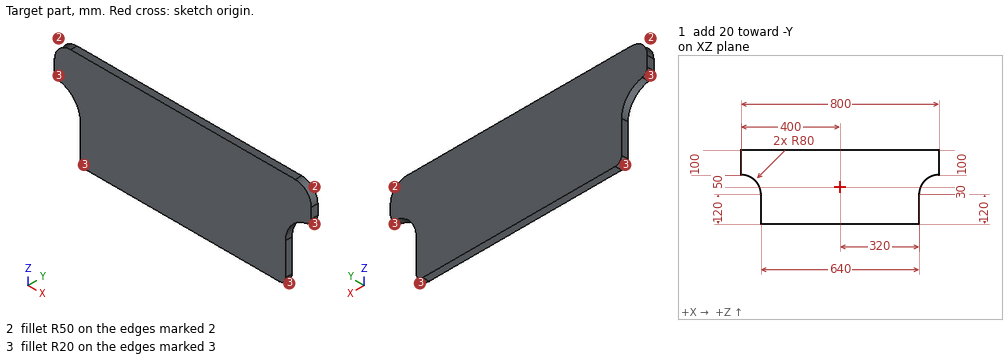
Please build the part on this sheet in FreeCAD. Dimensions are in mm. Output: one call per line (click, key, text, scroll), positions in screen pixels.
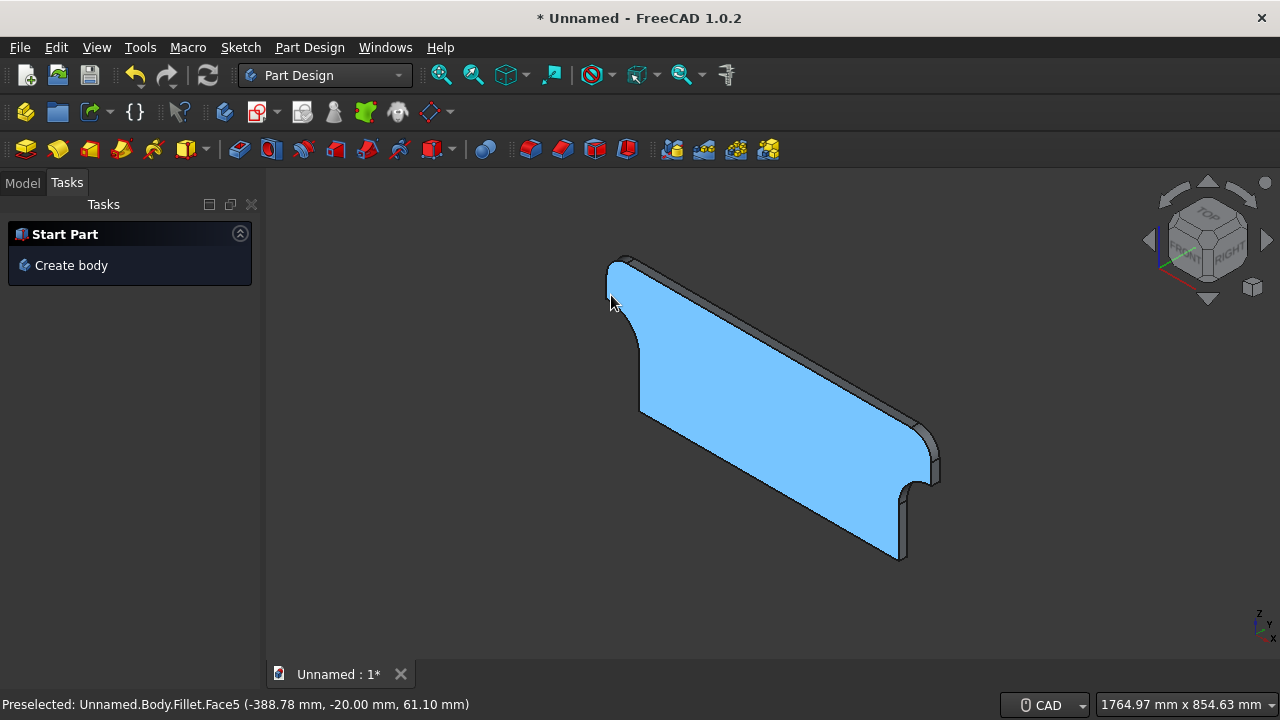
key(2)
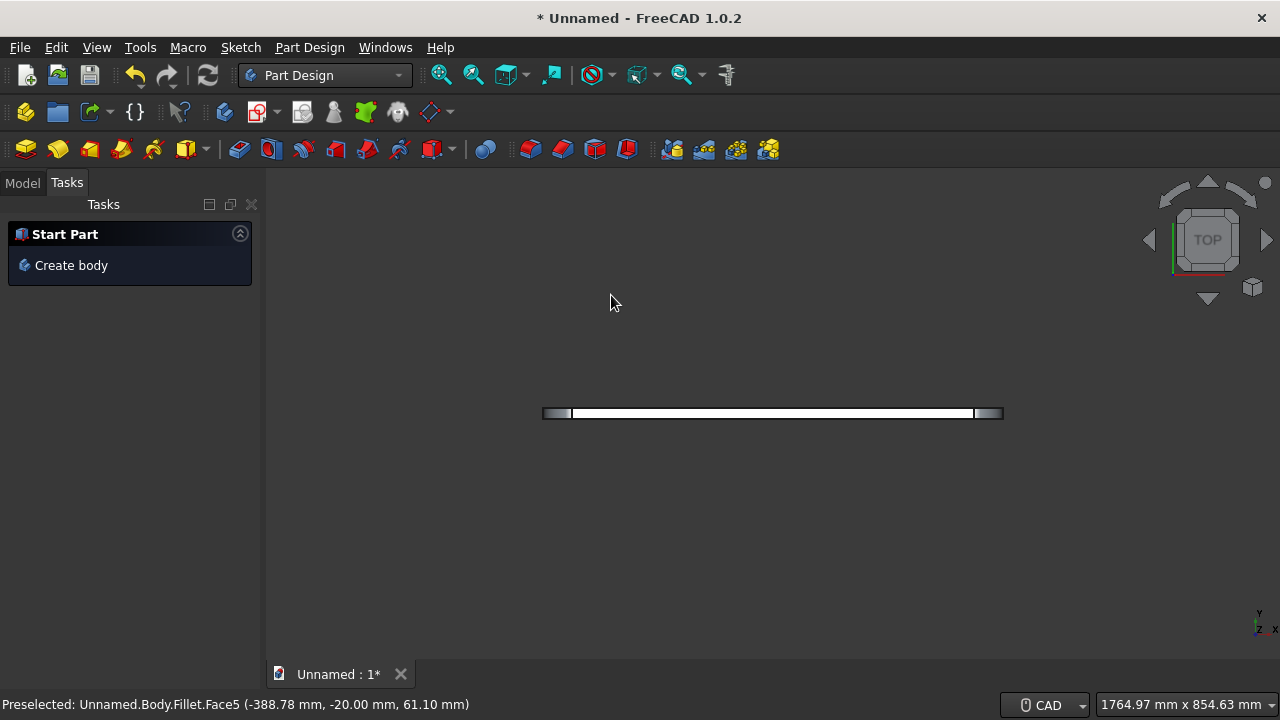
scroll(543, 412, up, 7)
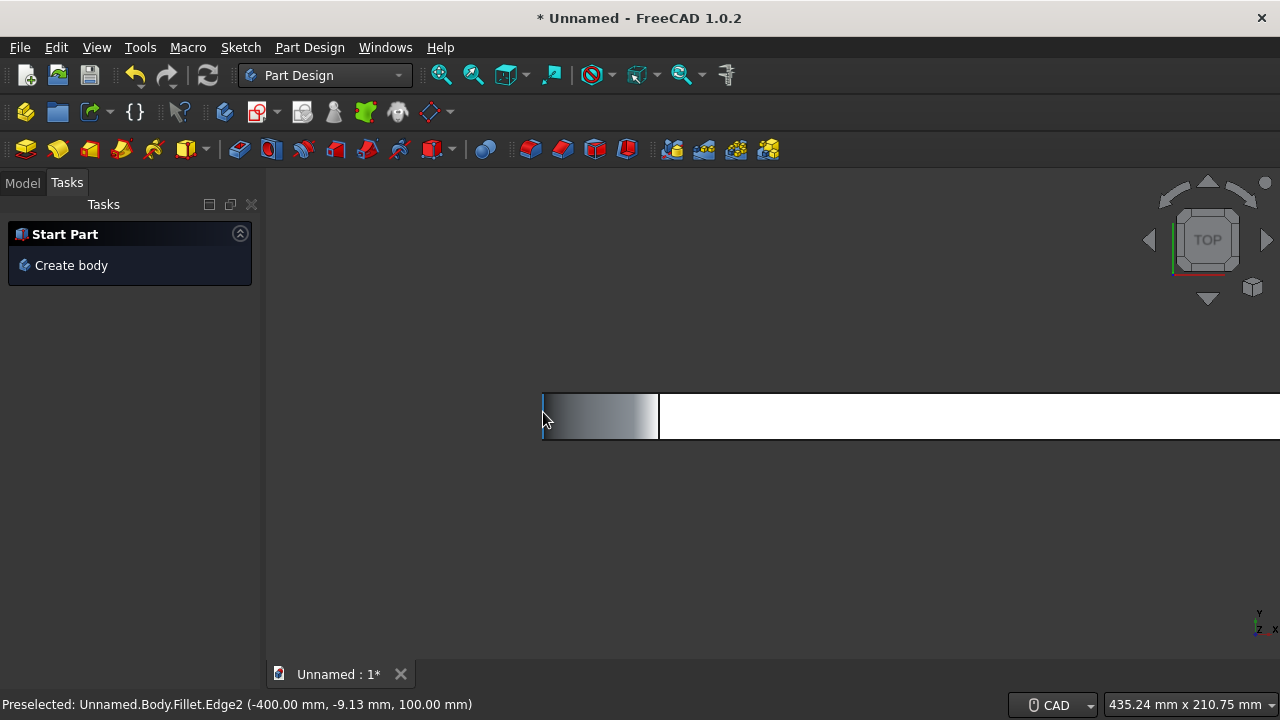
key(v)
key(f)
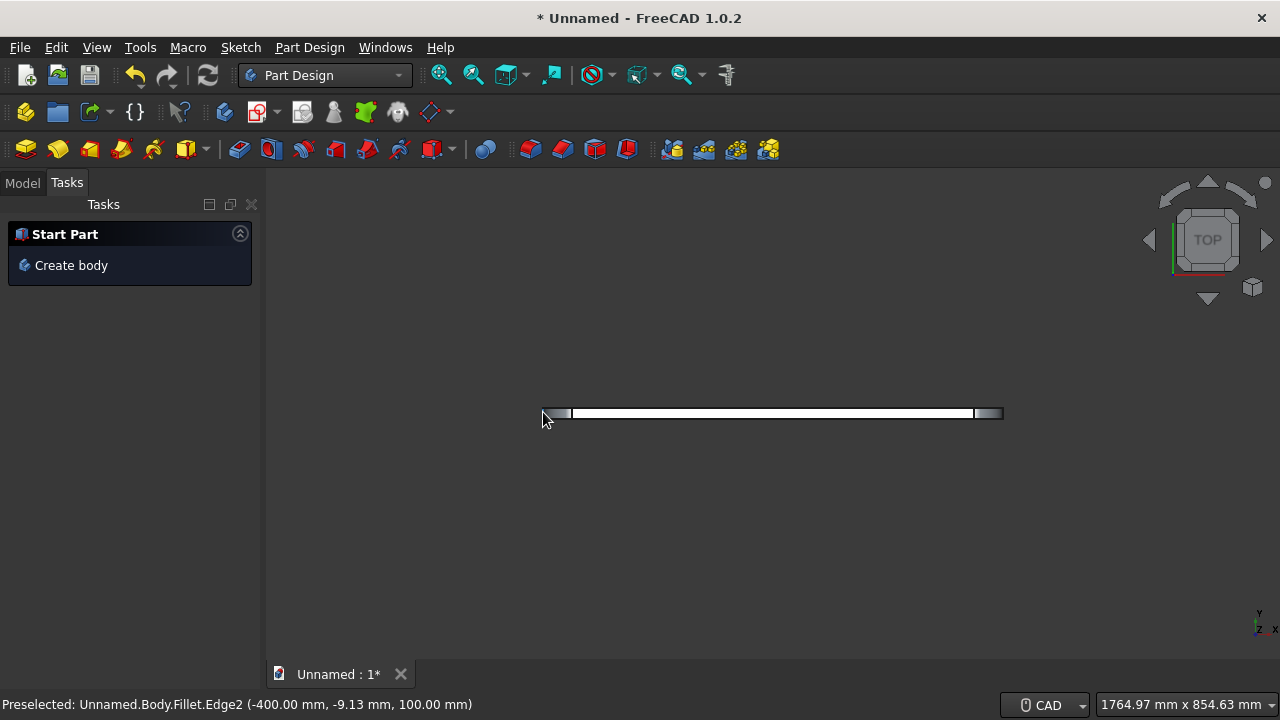
key(1)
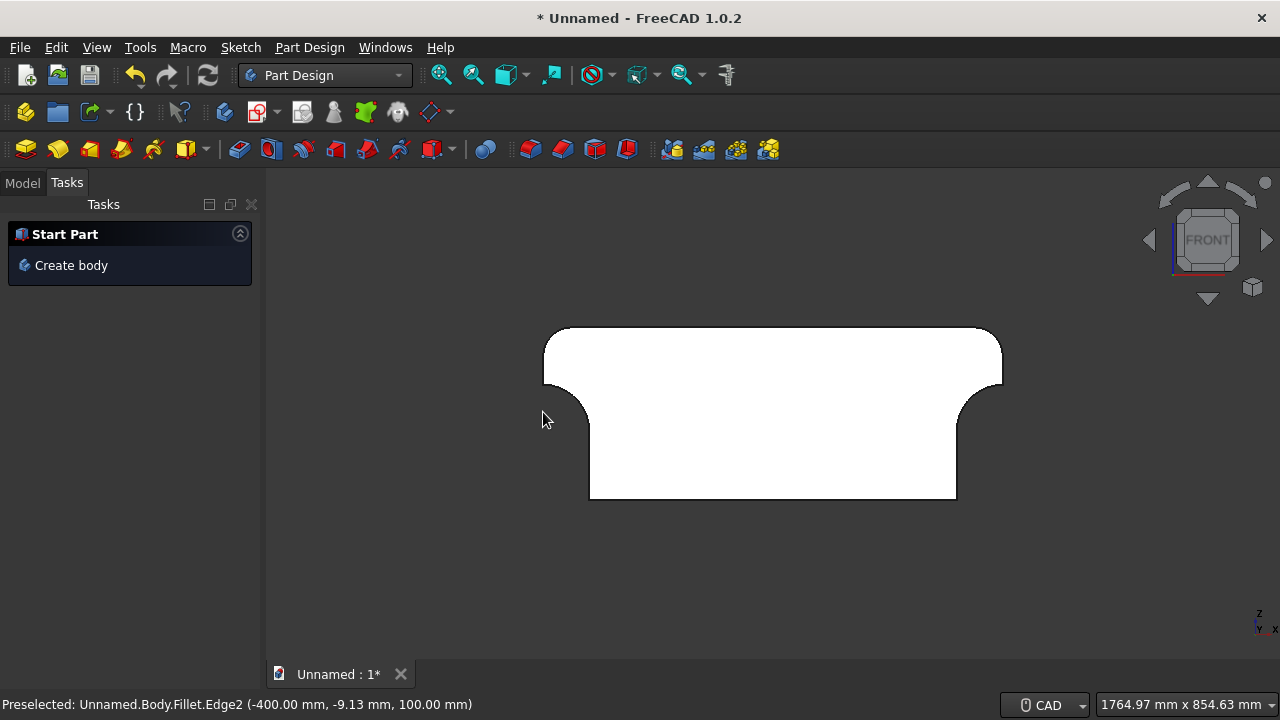
scroll(543, 384, up, 7)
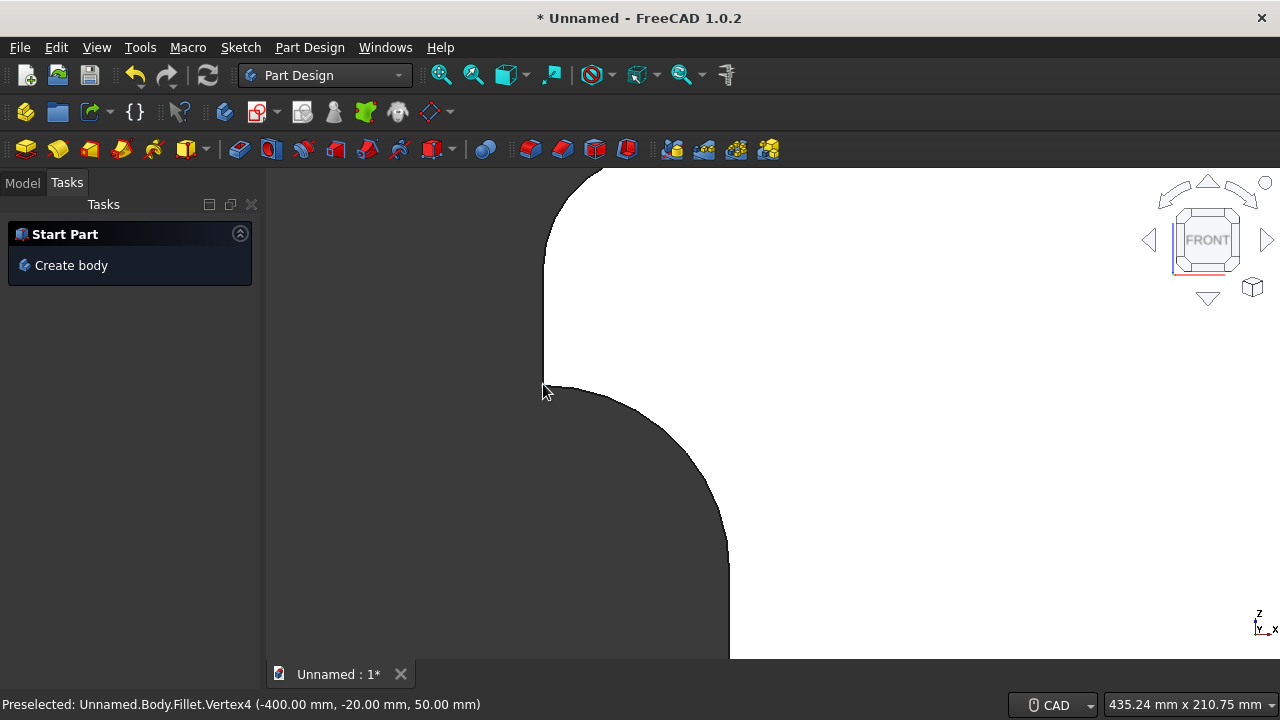
click(442, 76)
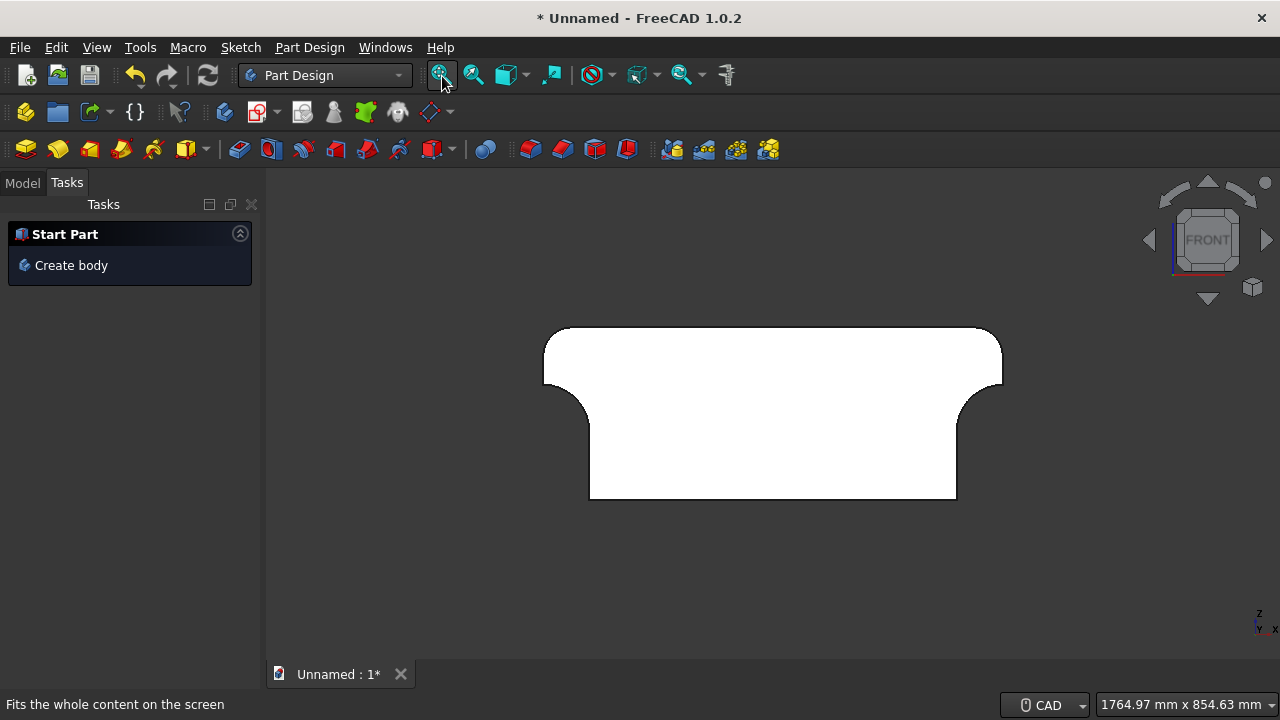
key(3)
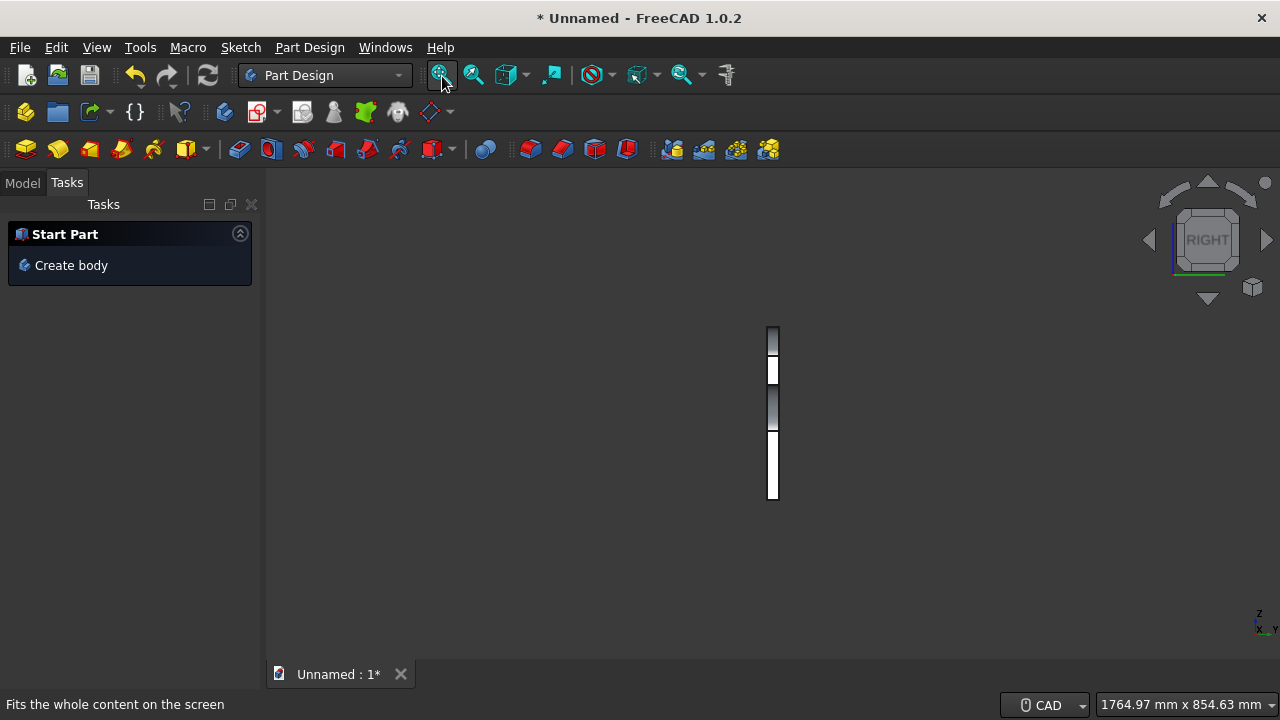
click(442, 76)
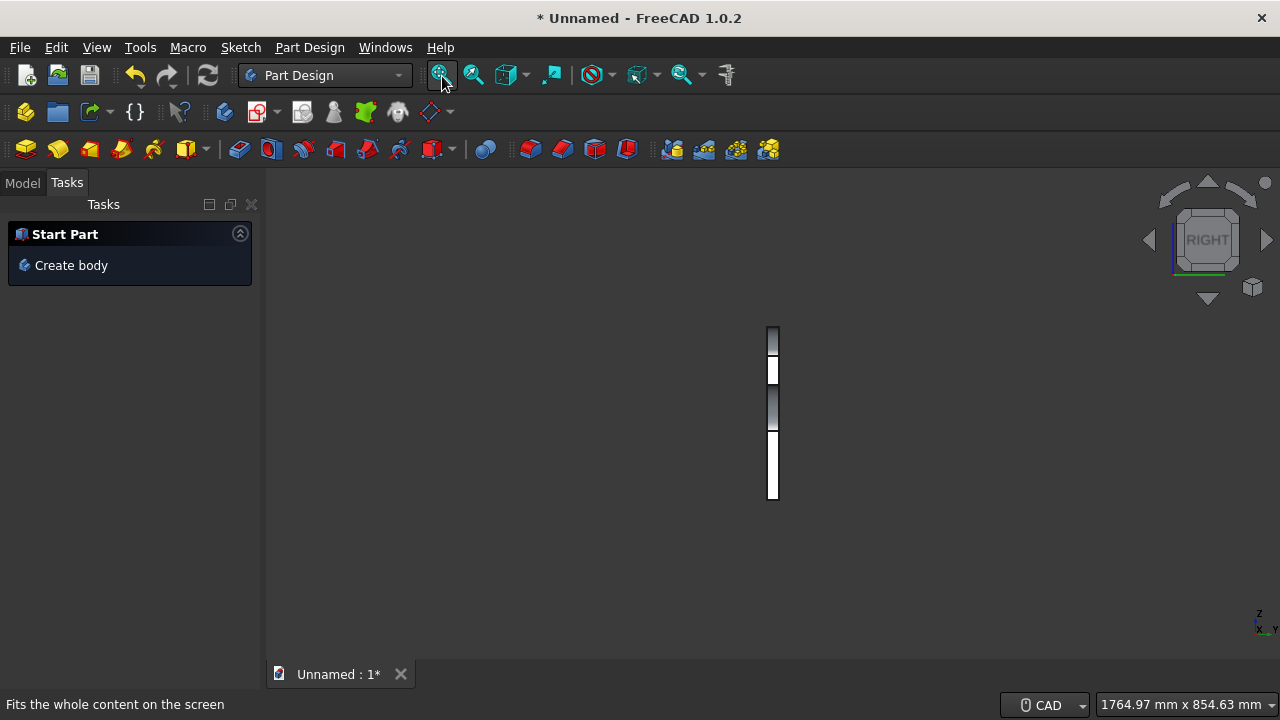
scroll(773, 384, up, 7)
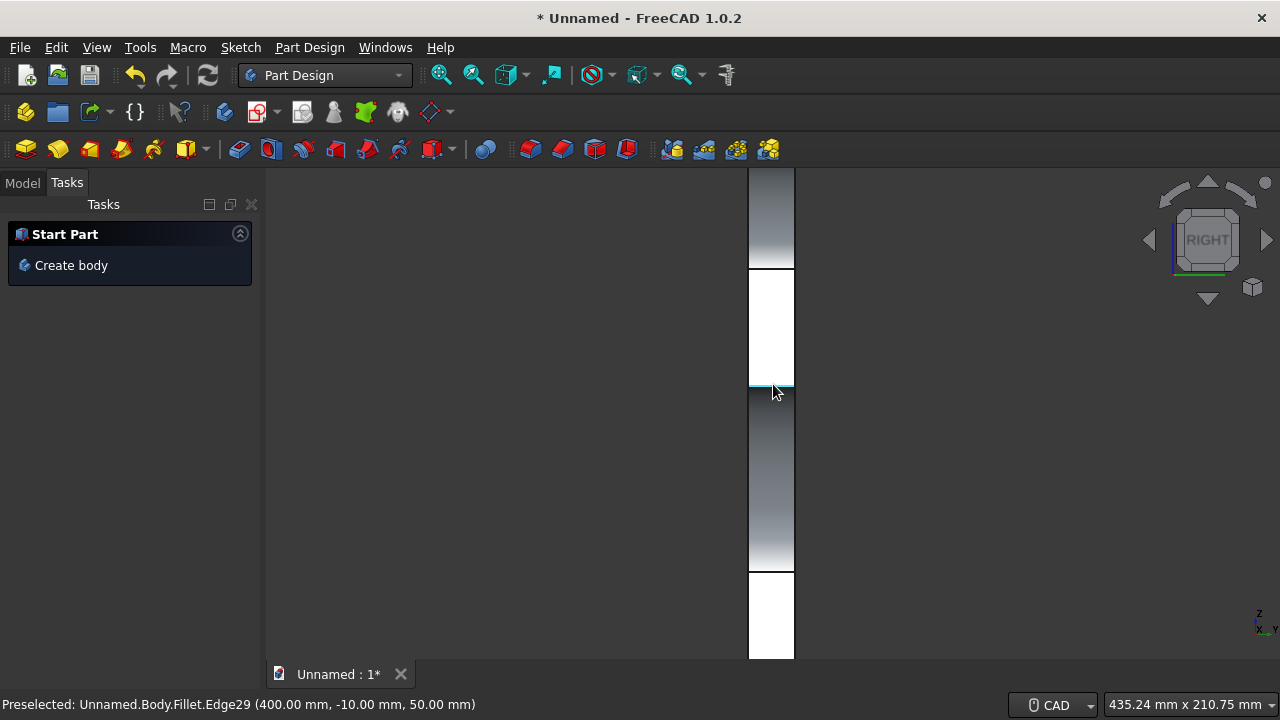
click(771, 385)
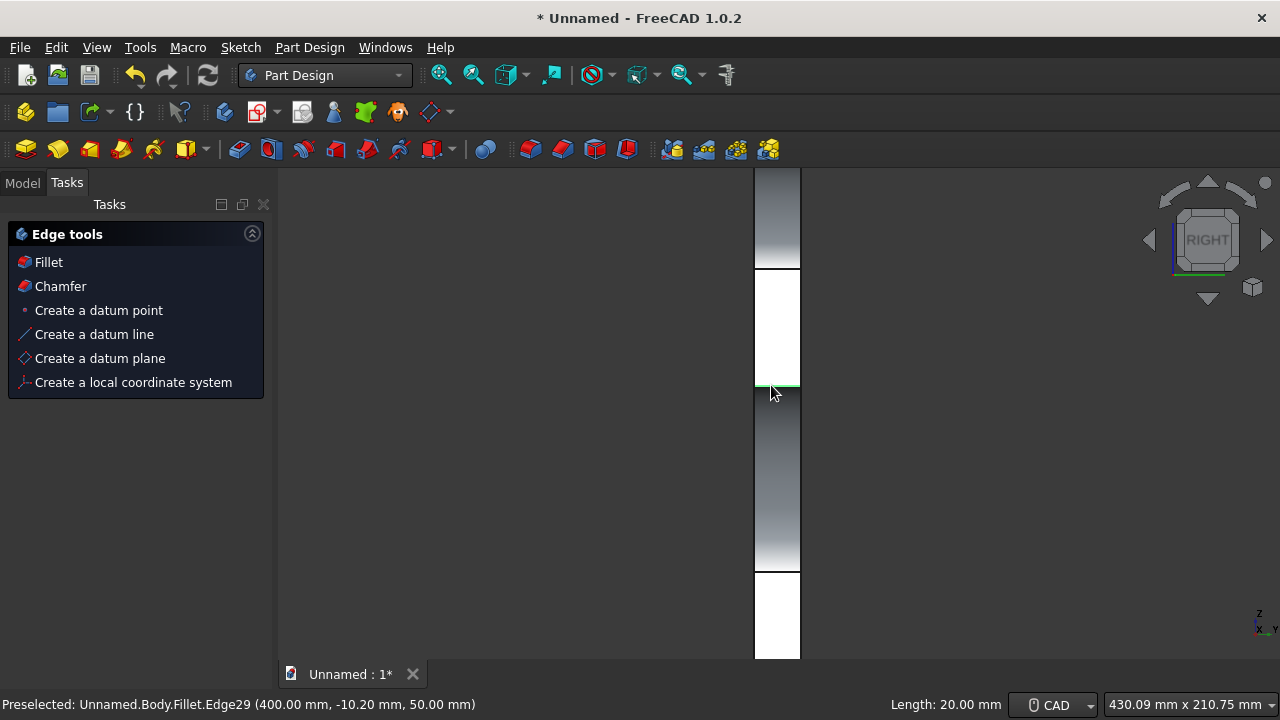
click(442, 76)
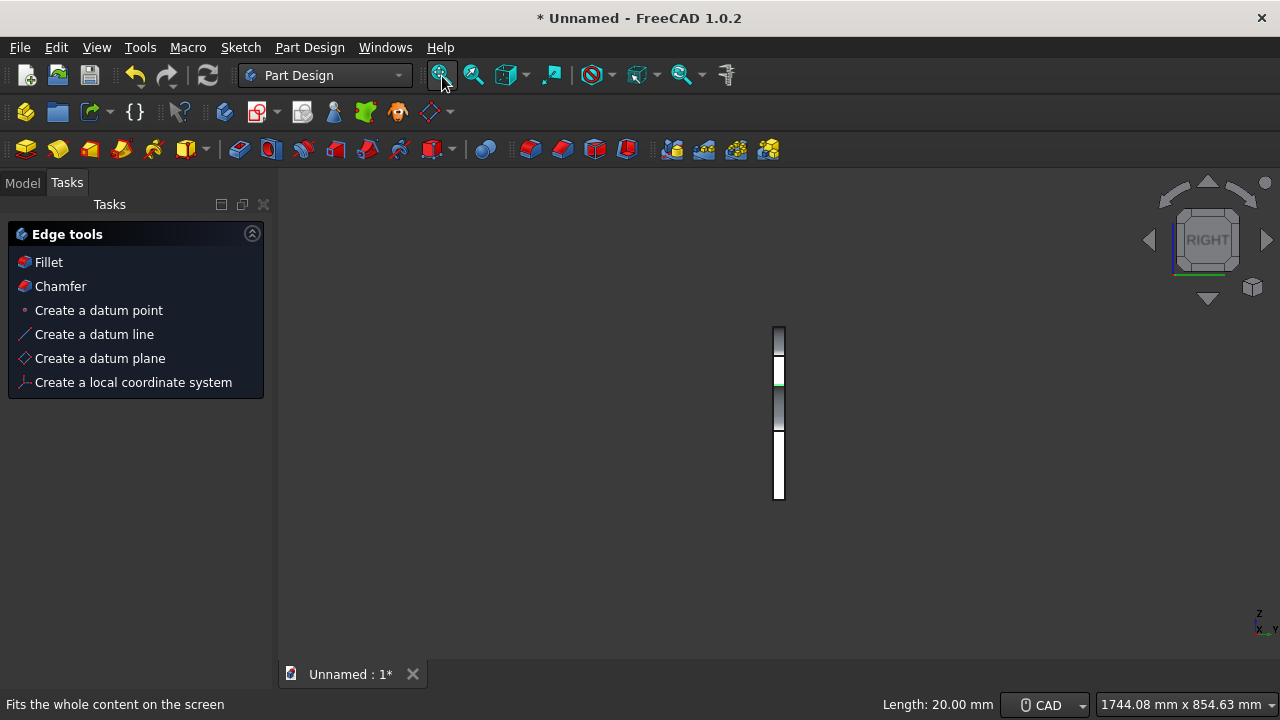
key(5)